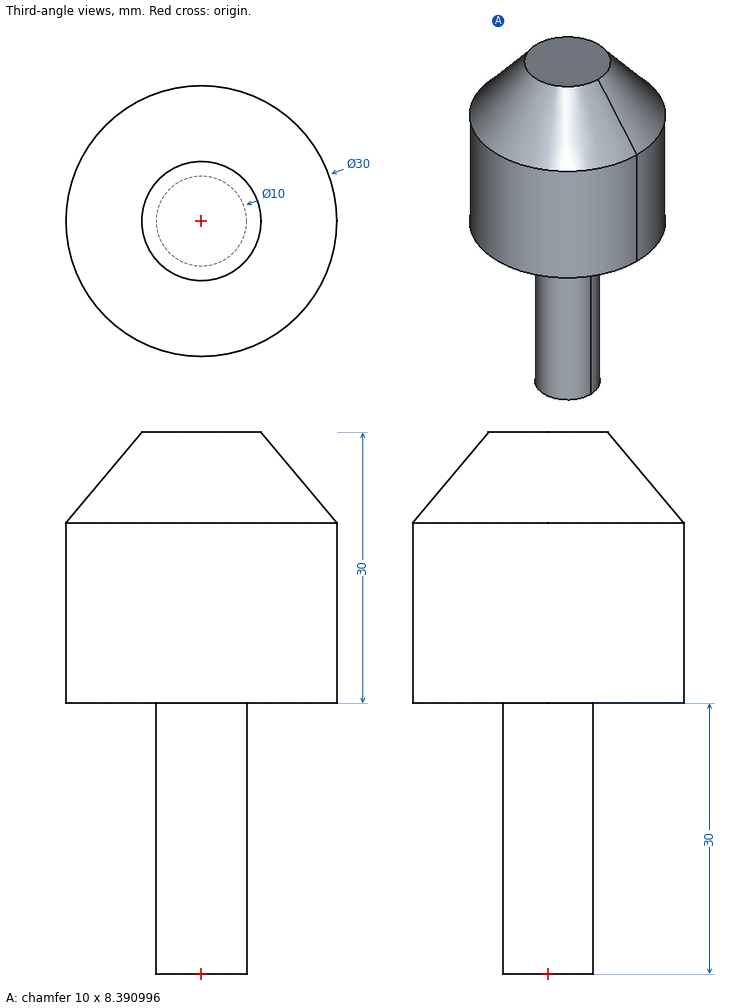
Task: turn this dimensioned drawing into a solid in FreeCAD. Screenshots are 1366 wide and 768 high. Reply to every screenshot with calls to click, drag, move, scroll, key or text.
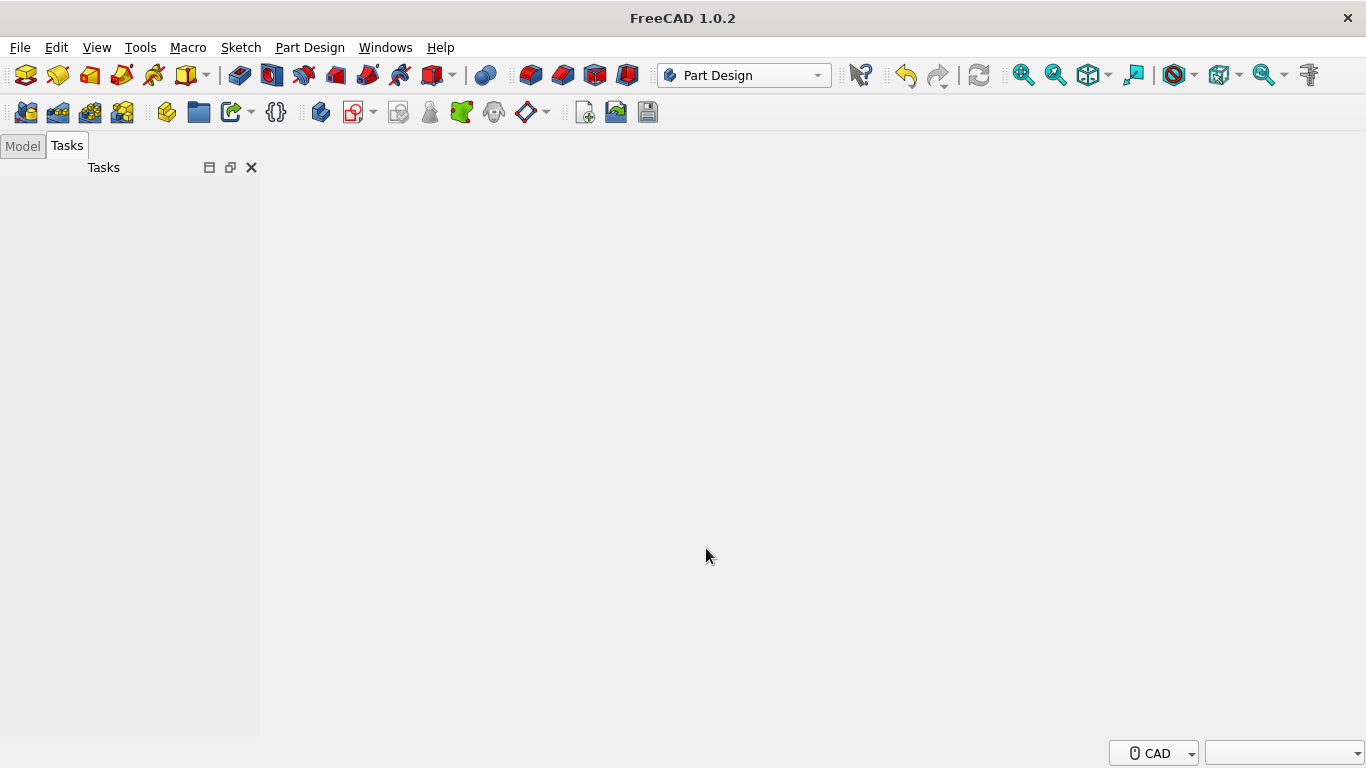
click(584, 112)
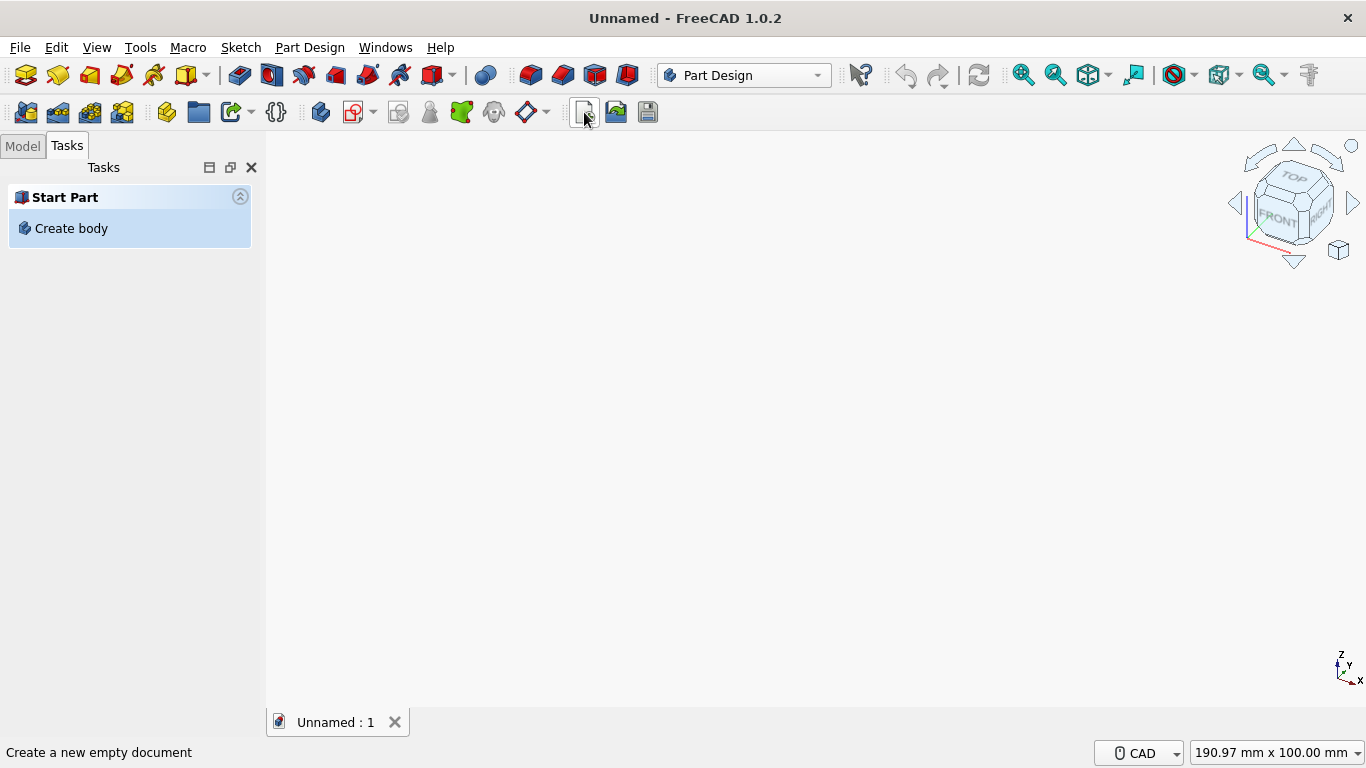
click(354, 112)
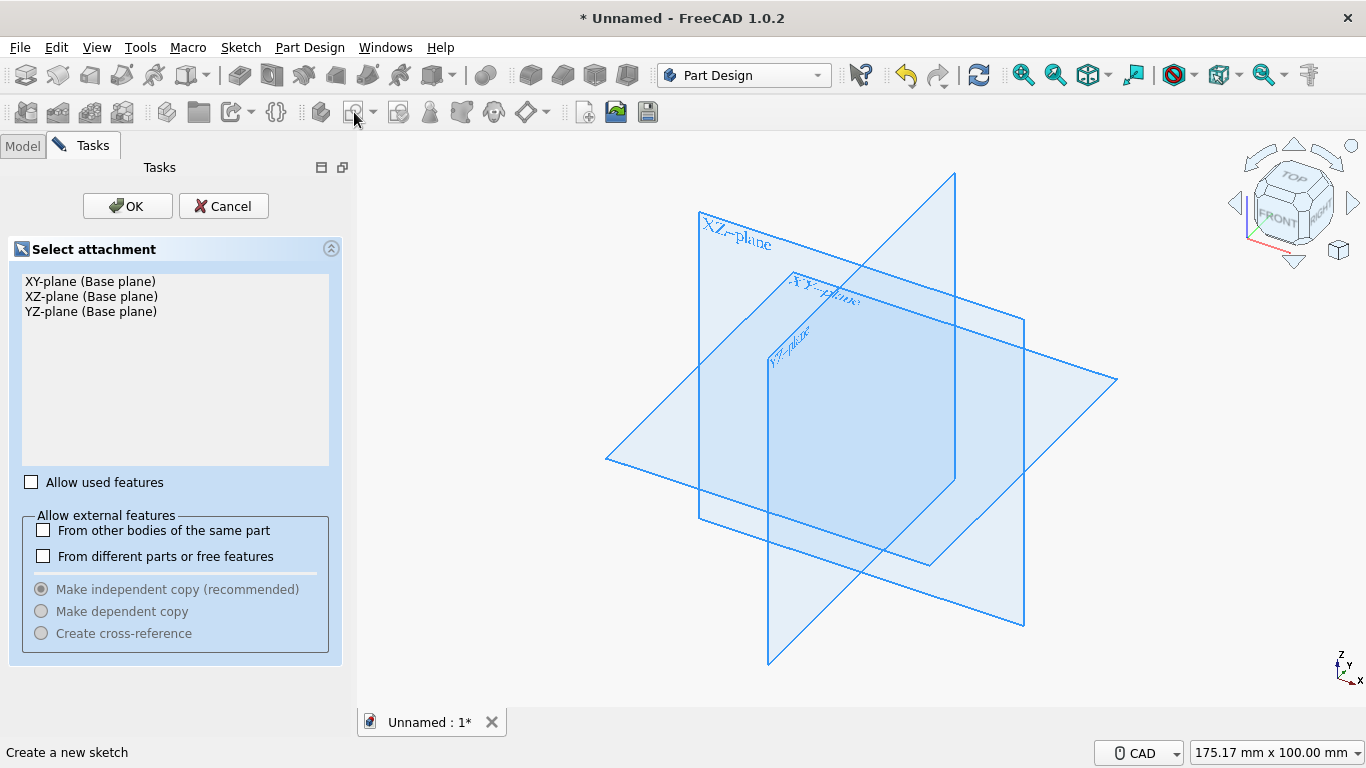
click(82, 282)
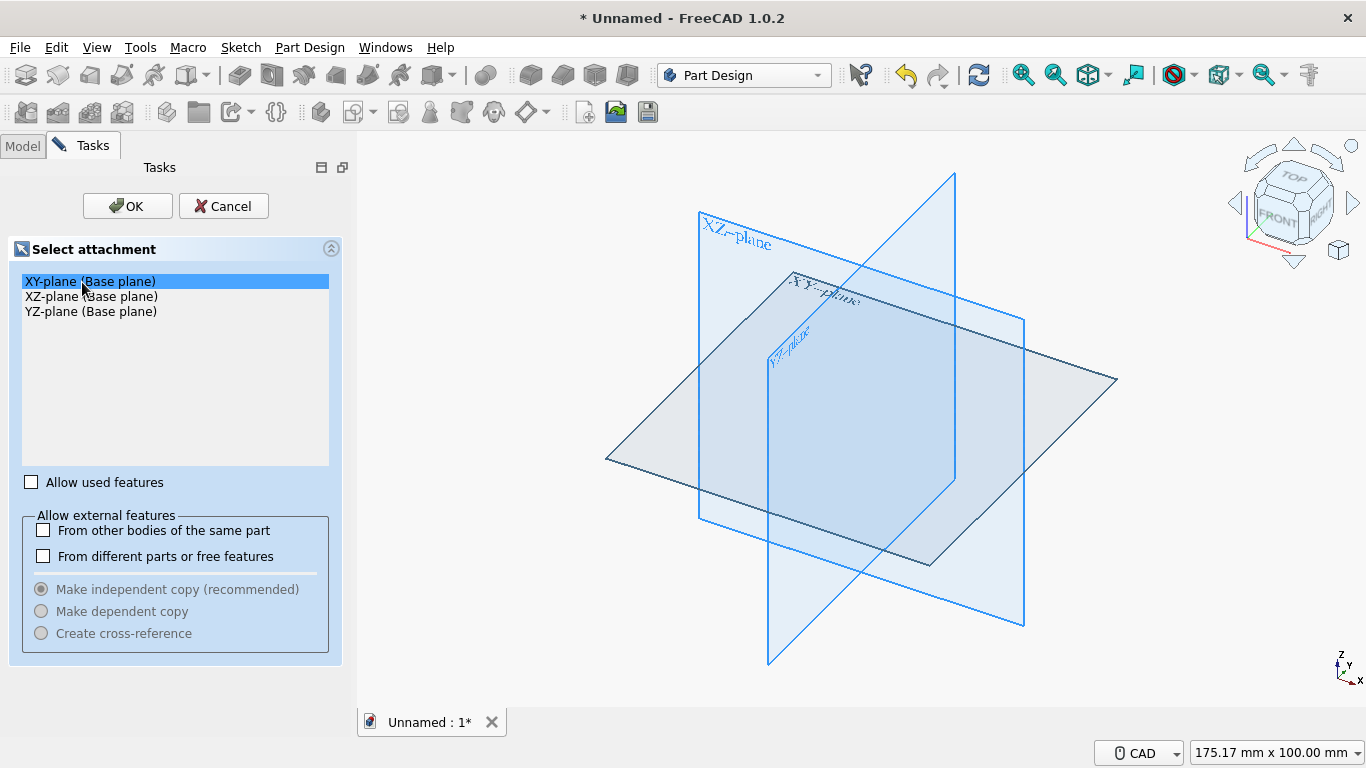
click(128, 206)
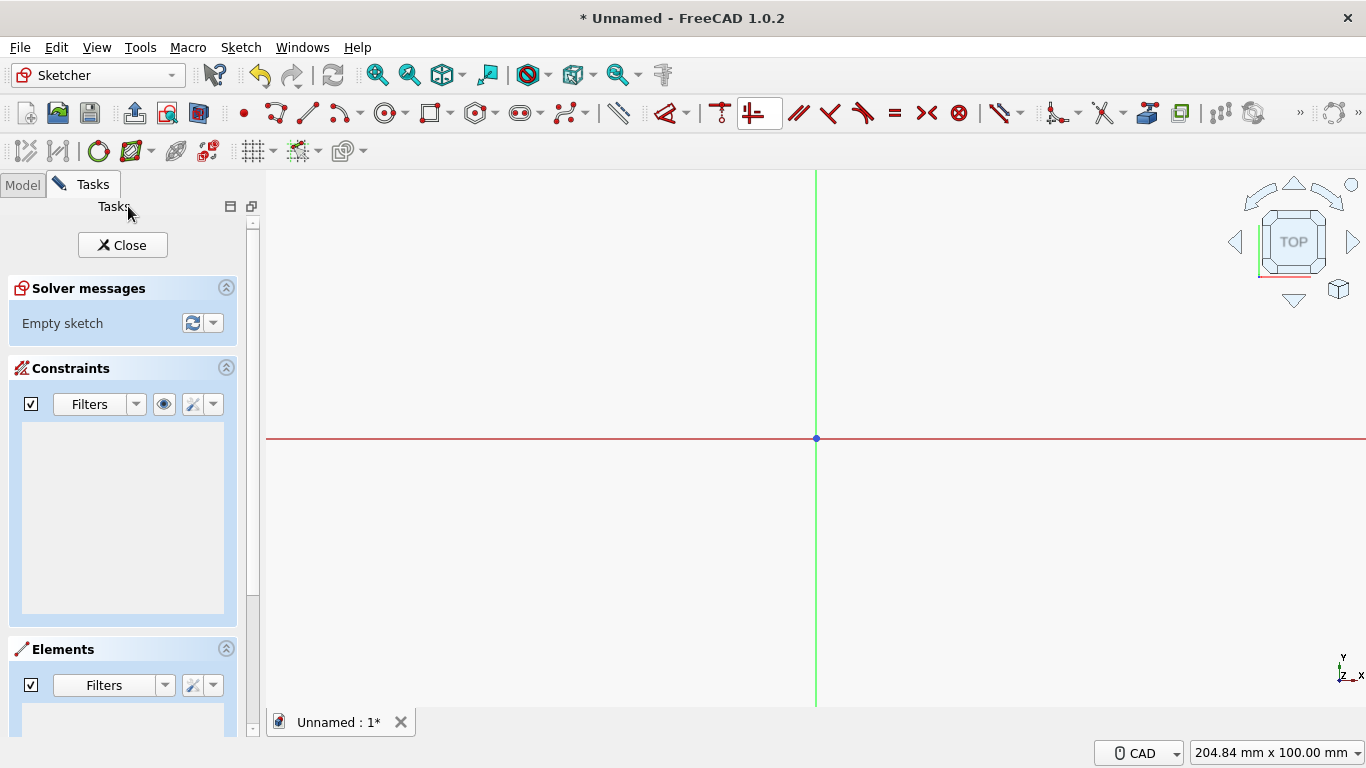
scroll(830, 438, up, 9)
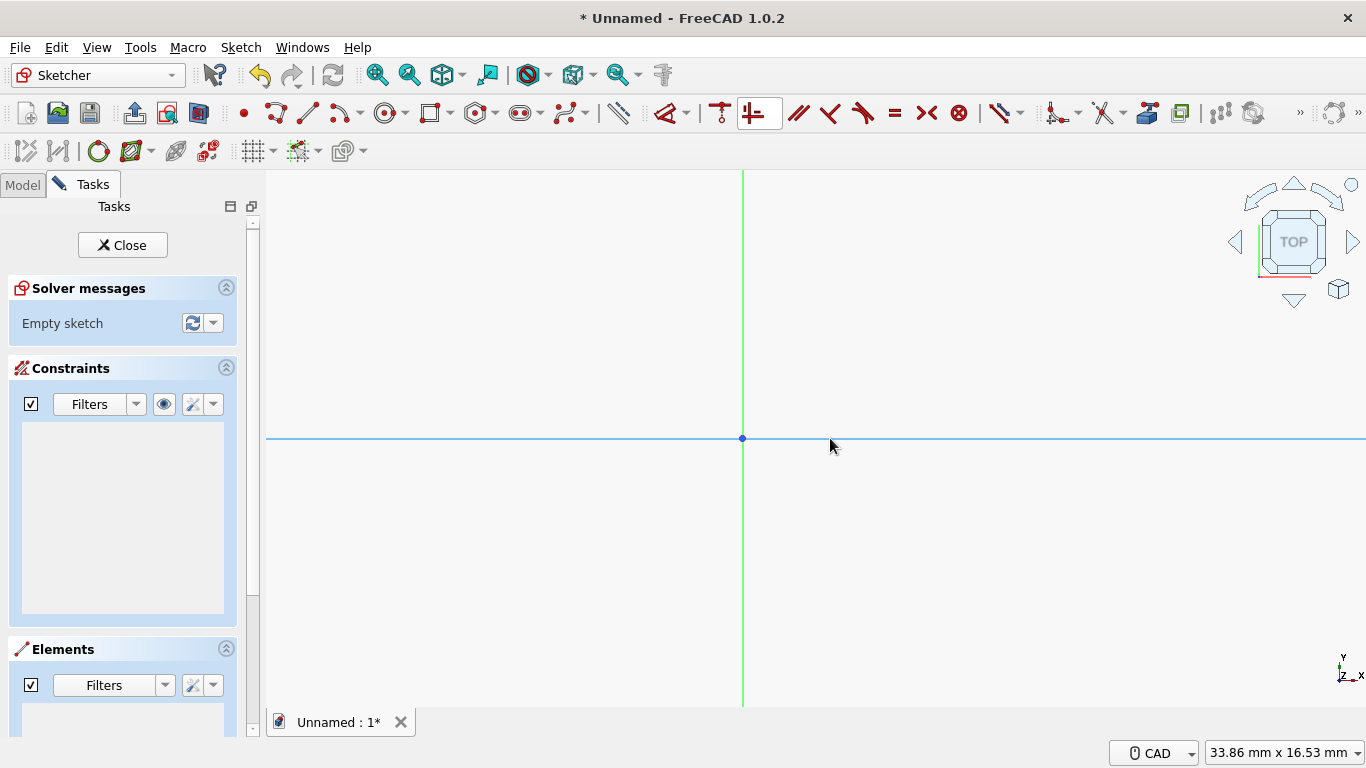
click(386, 114)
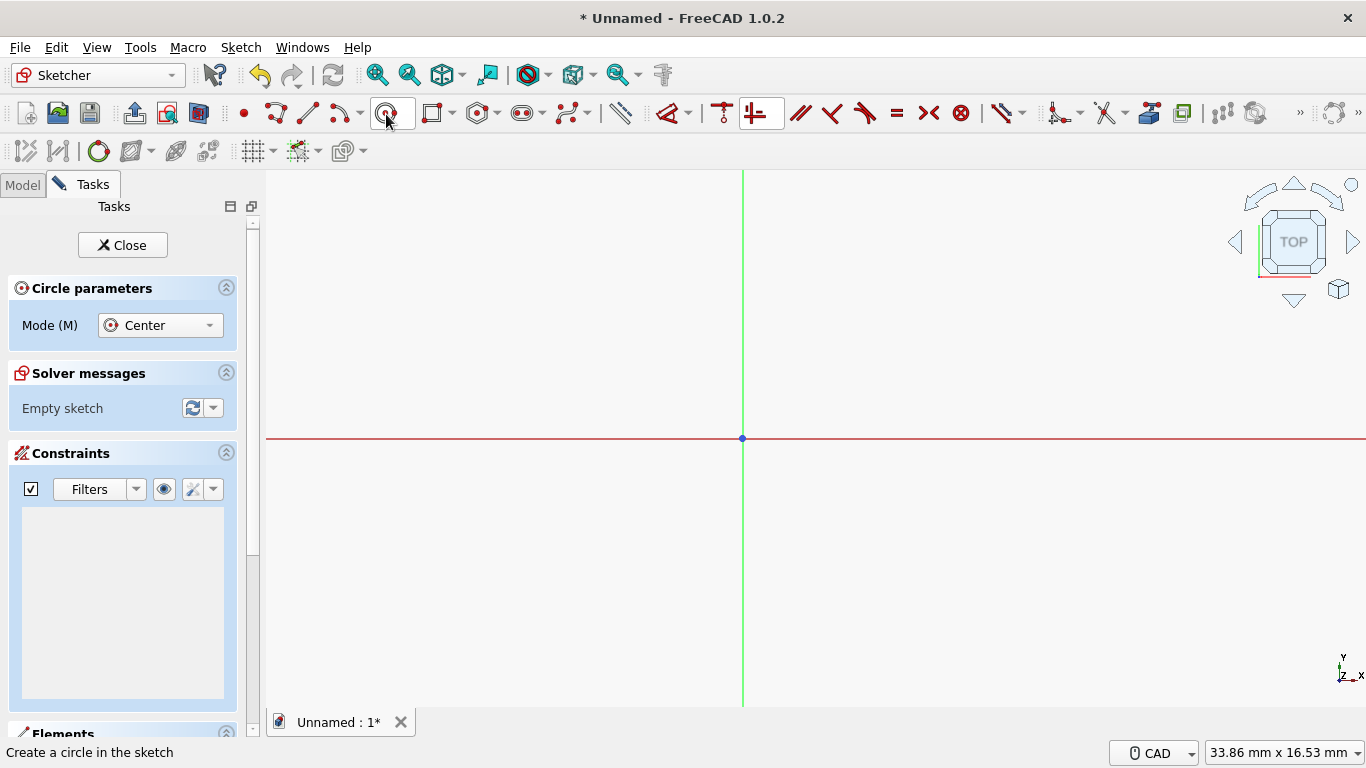
click(743, 438)
click(858, 324)
key(Escape)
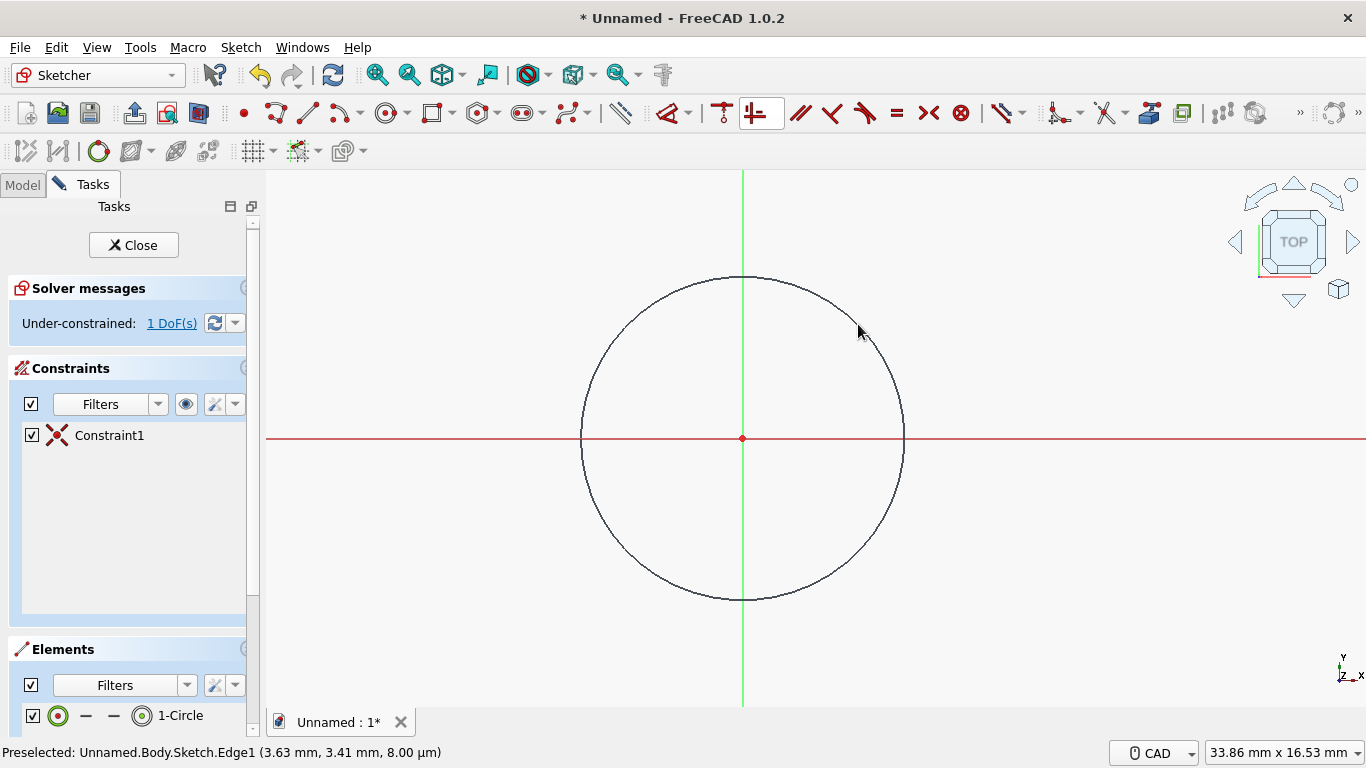
click(668, 114)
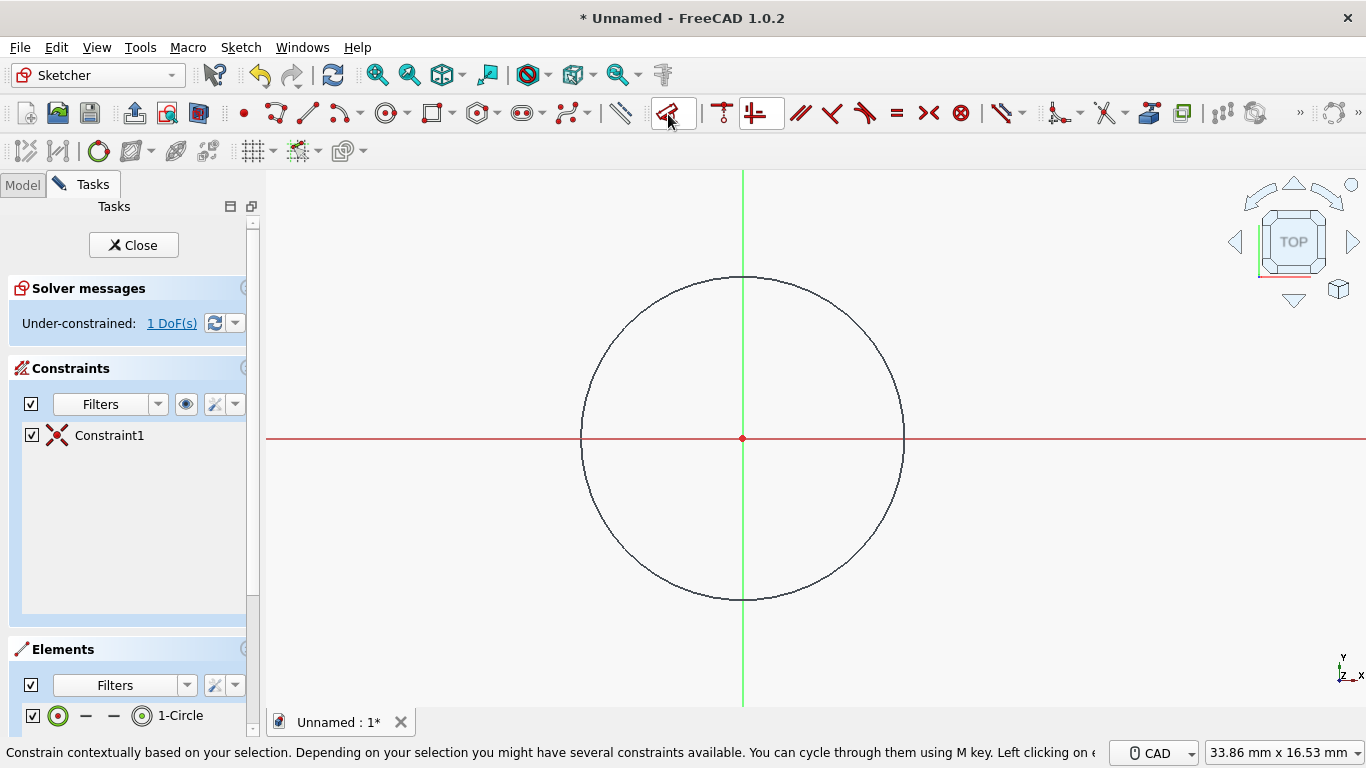
click(857, 324)
click(880, 301)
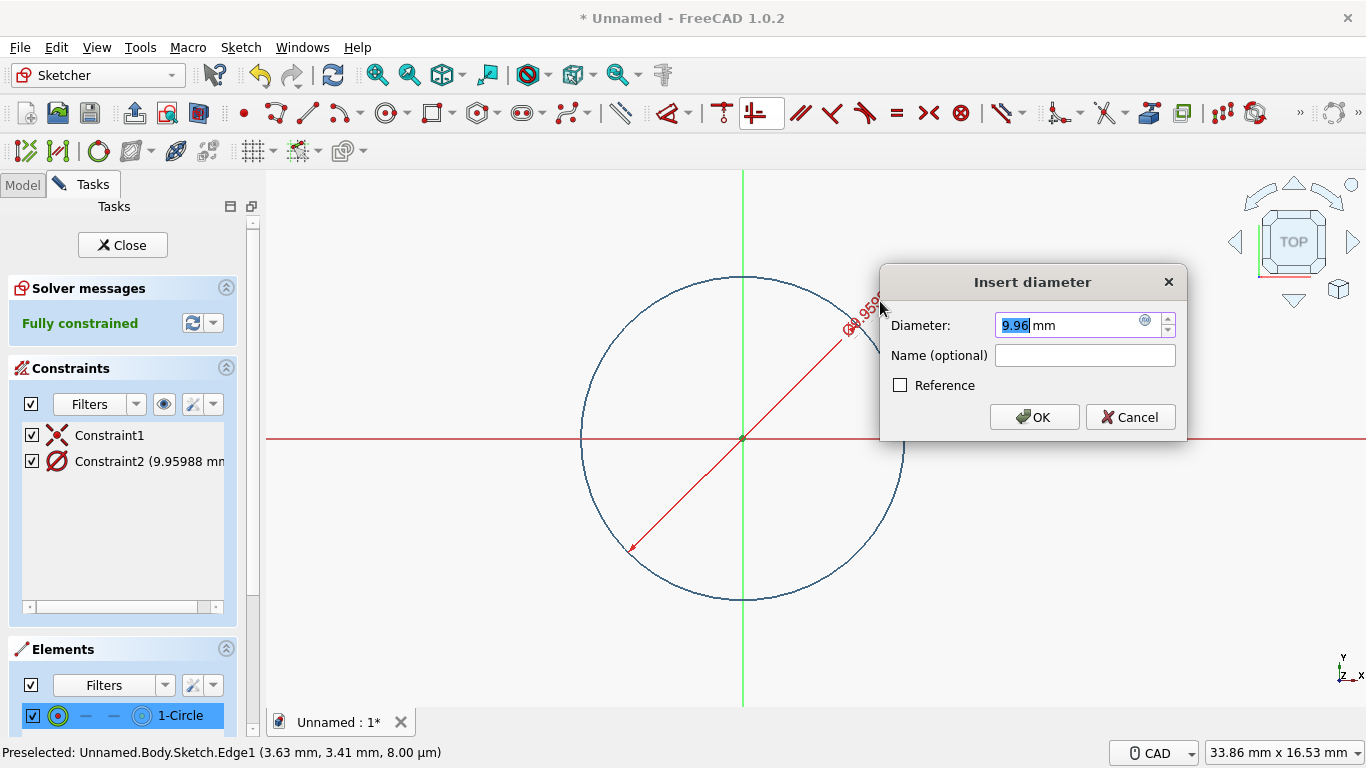
text(10)
key(Return)
key(Escape)